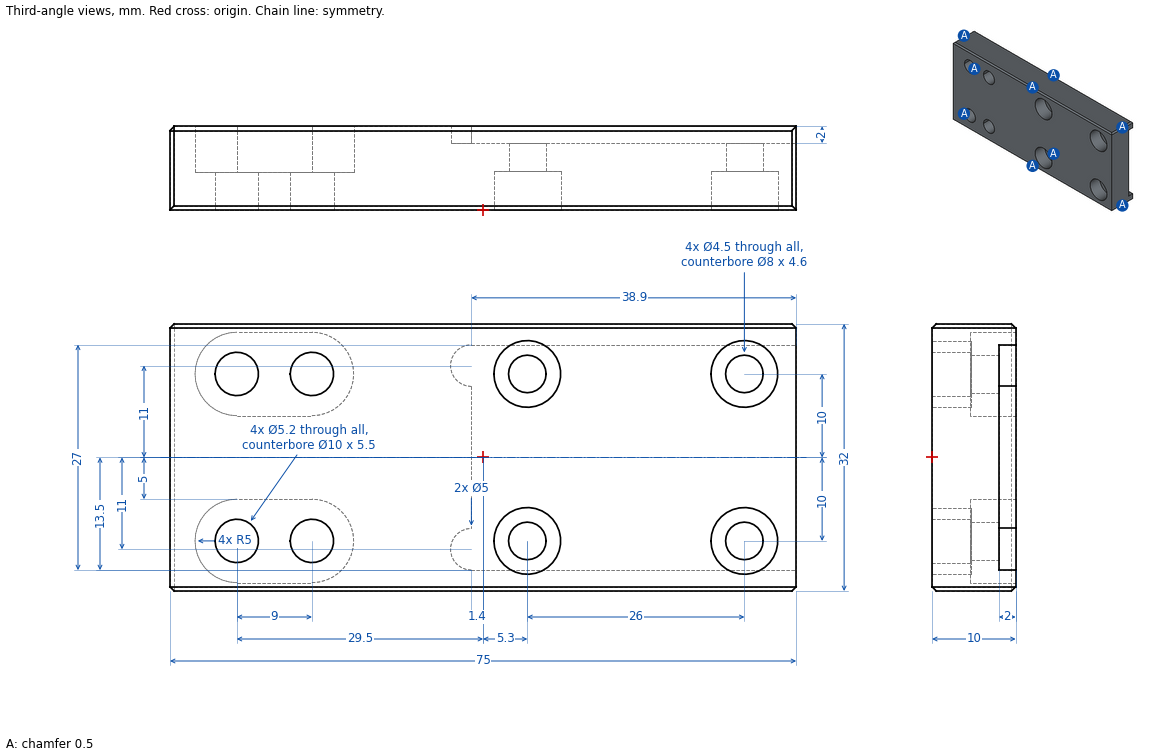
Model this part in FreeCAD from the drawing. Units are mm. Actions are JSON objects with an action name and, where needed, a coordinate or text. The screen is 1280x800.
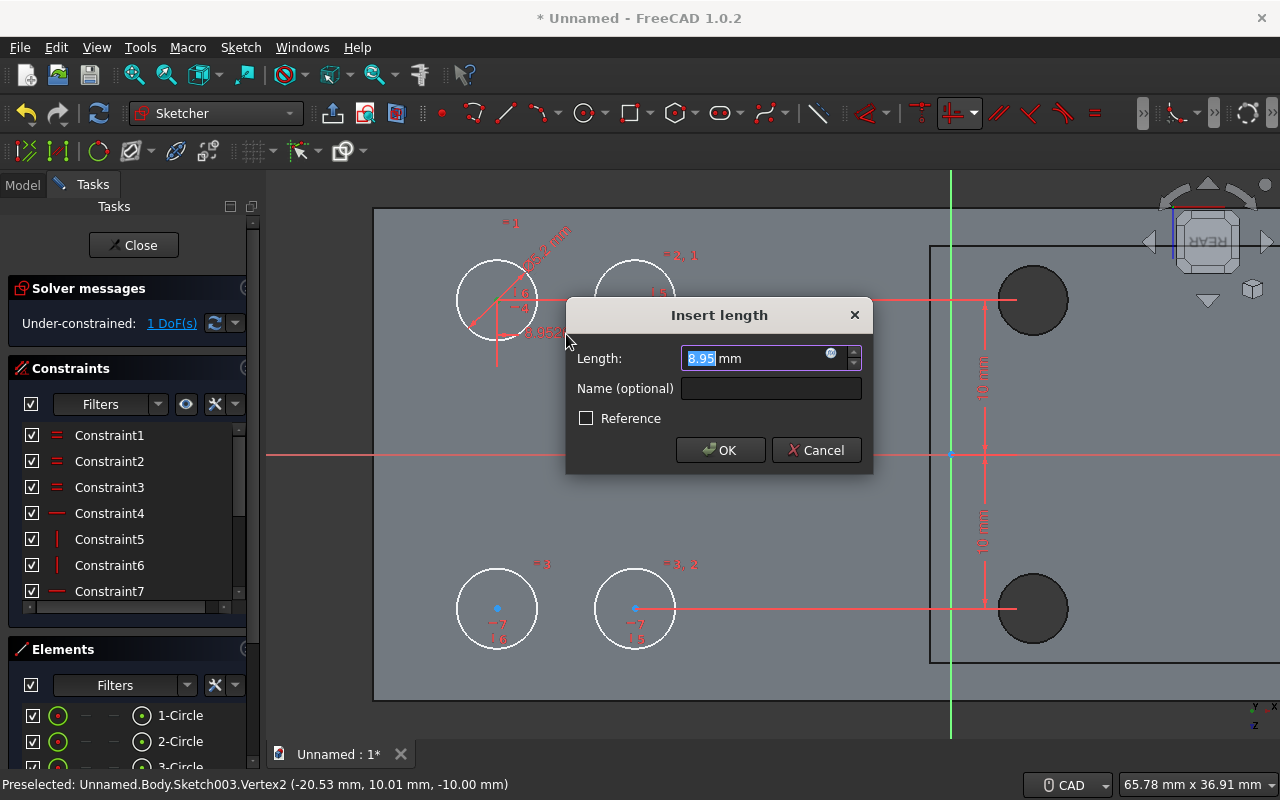
{"action": "type", "text": "9"}
{"action": "key", "text": "Return"}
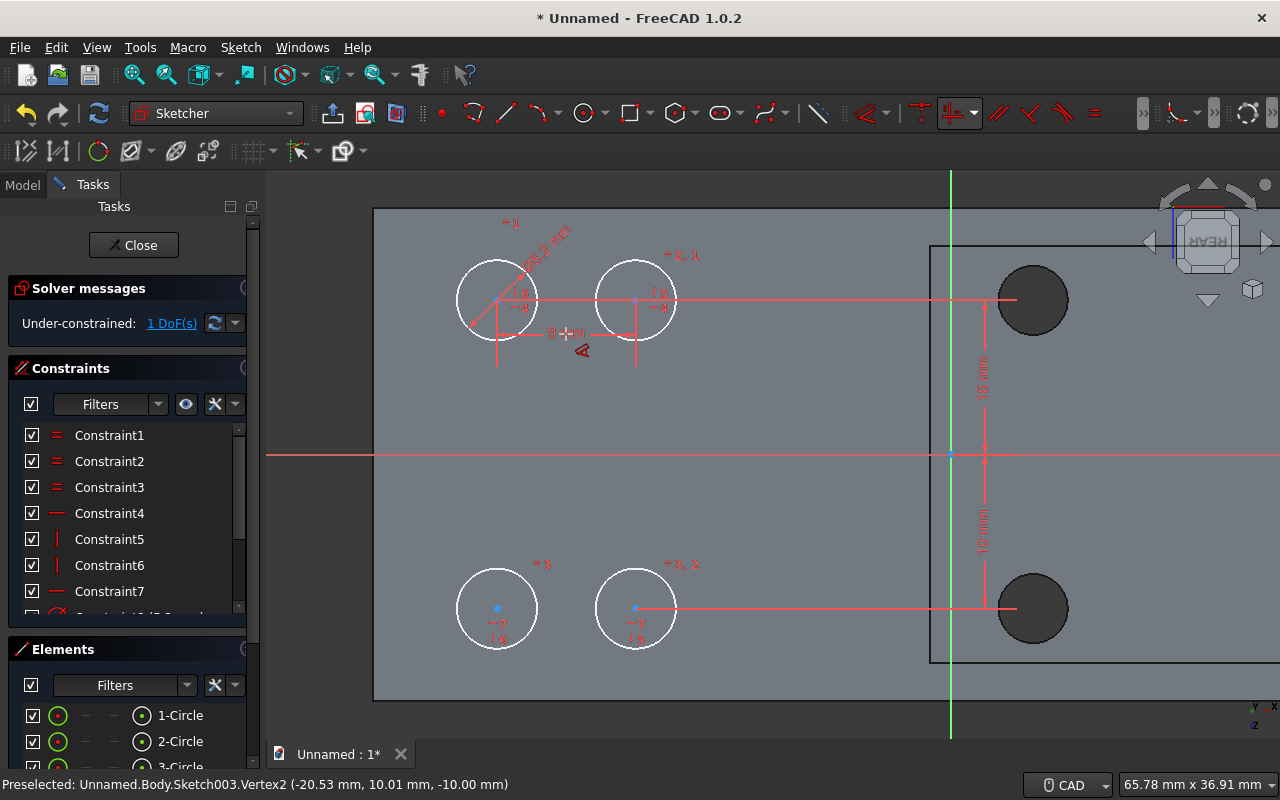
{"action": "left_click", "coordinate": [497, 300]}
{"action": "left_click", "coordinate": [724, 266]}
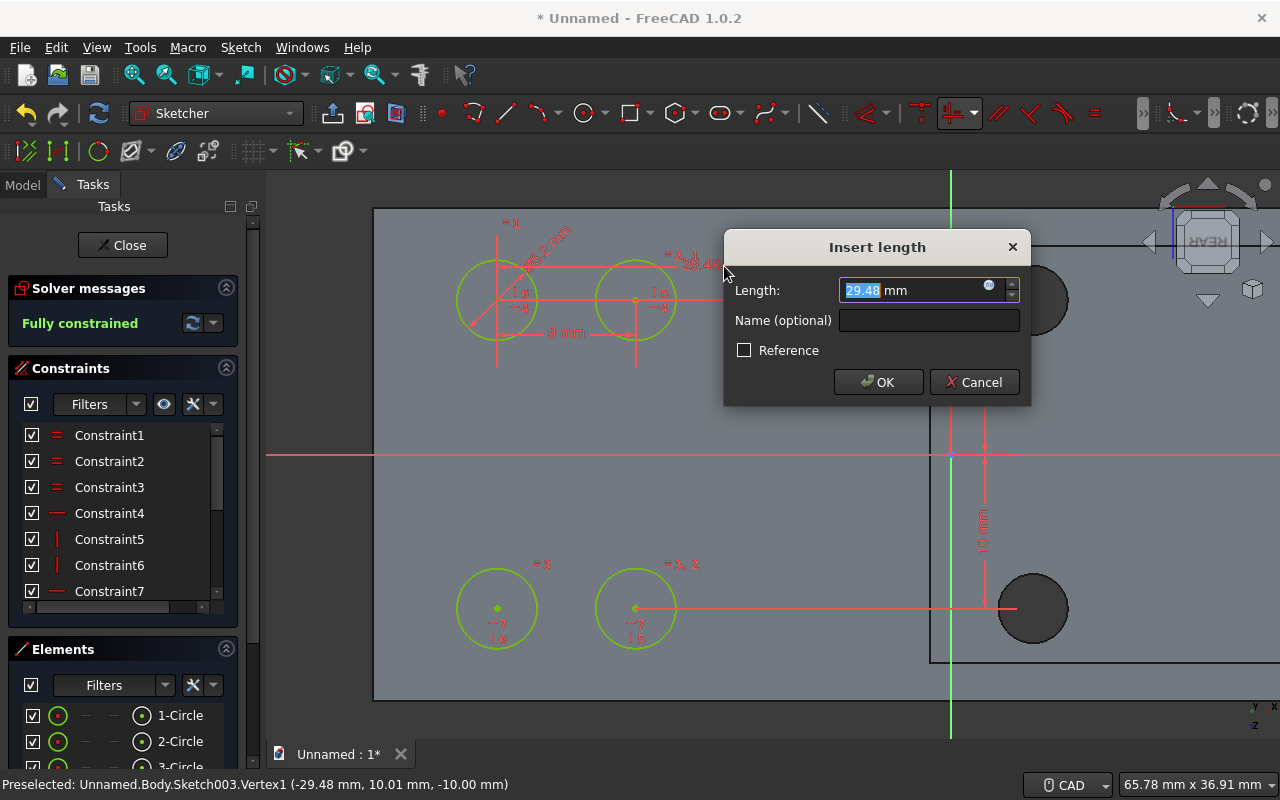
{"action": "type", "text": "29.5"}
{"action": "key", "text": "Return"}
{"action": "key", "text": "Escape"}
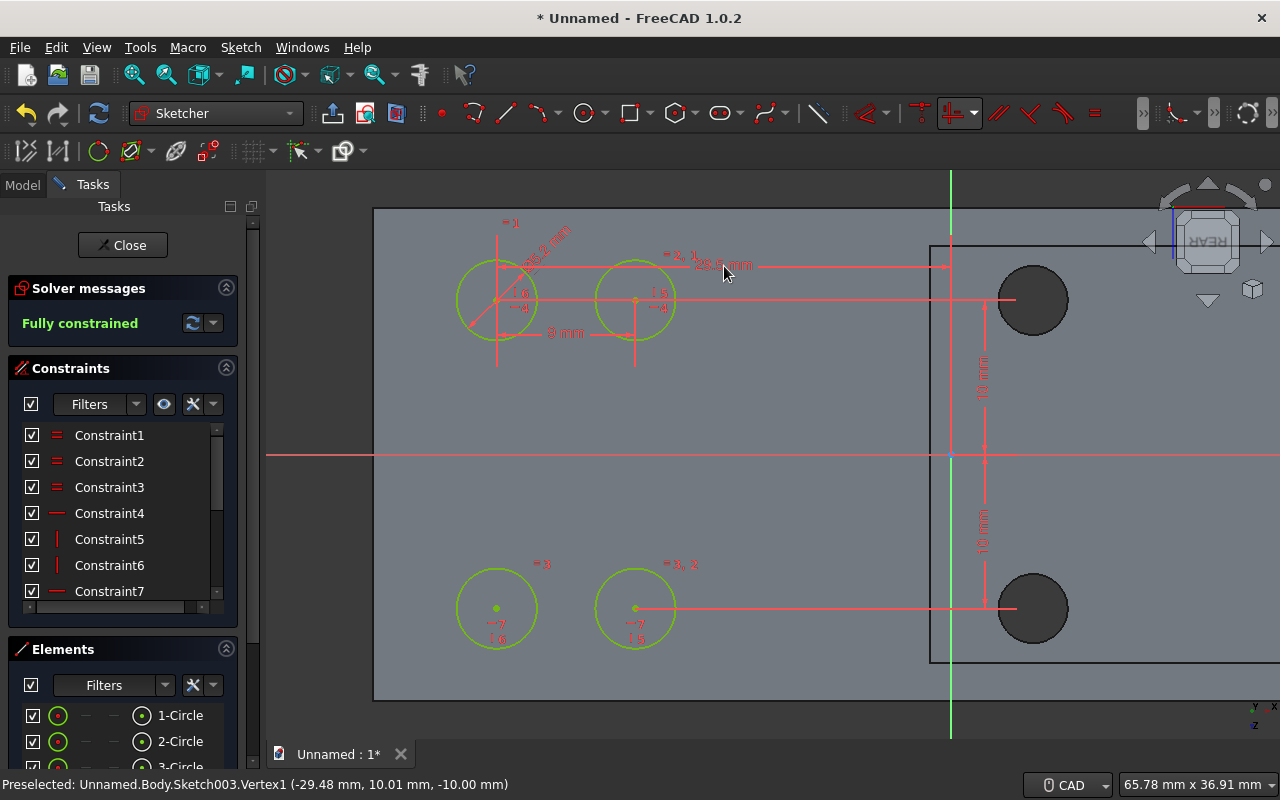
{"action": "left_click", "coordinate": [123, 245]}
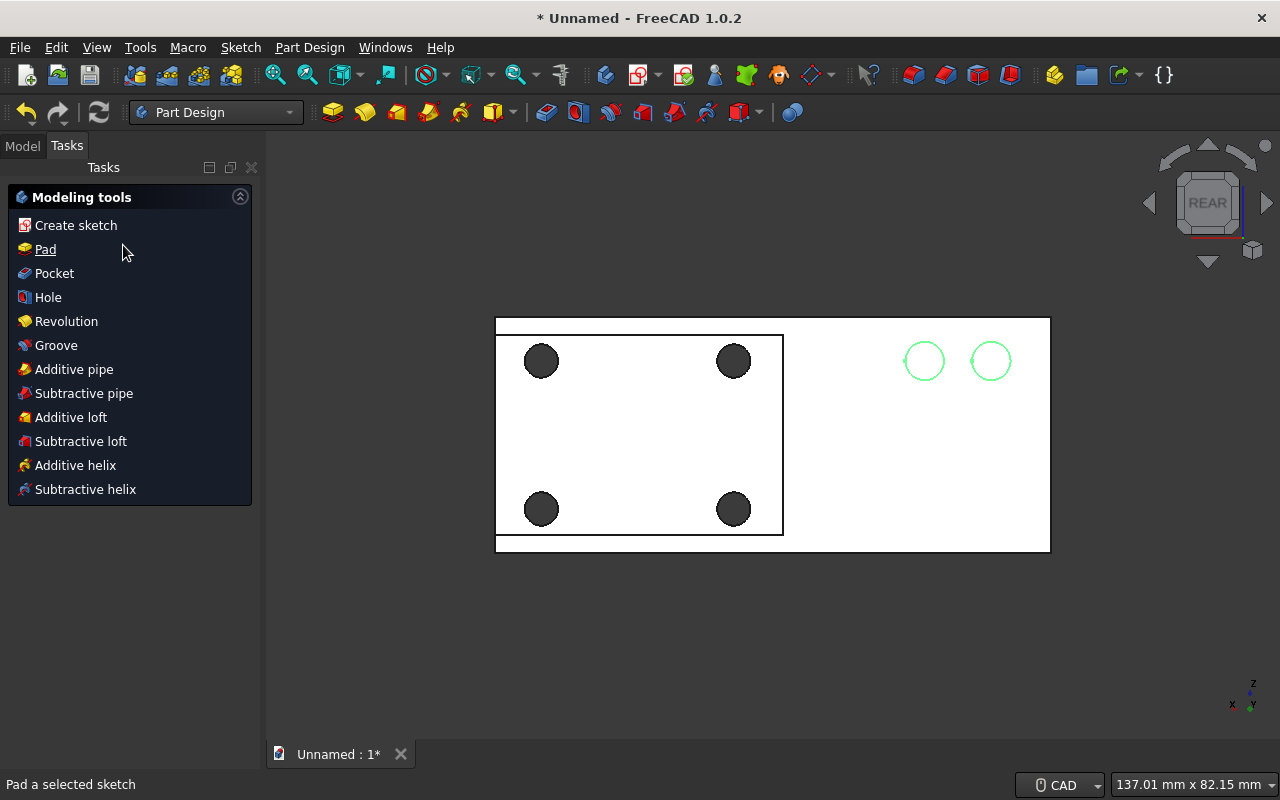
{"action": "left_click", "coordinate": [580, 112]}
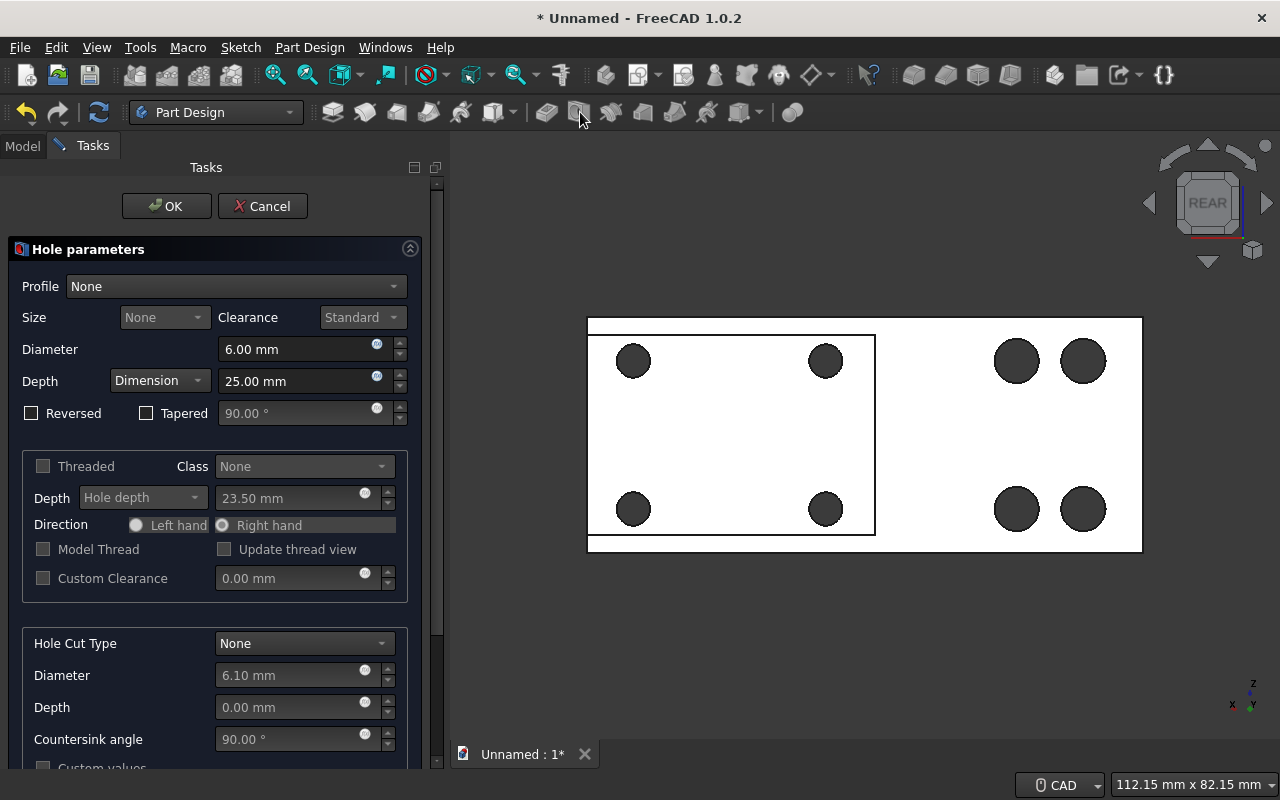
{"action": "triple_click", "coordinate": [305, 349]}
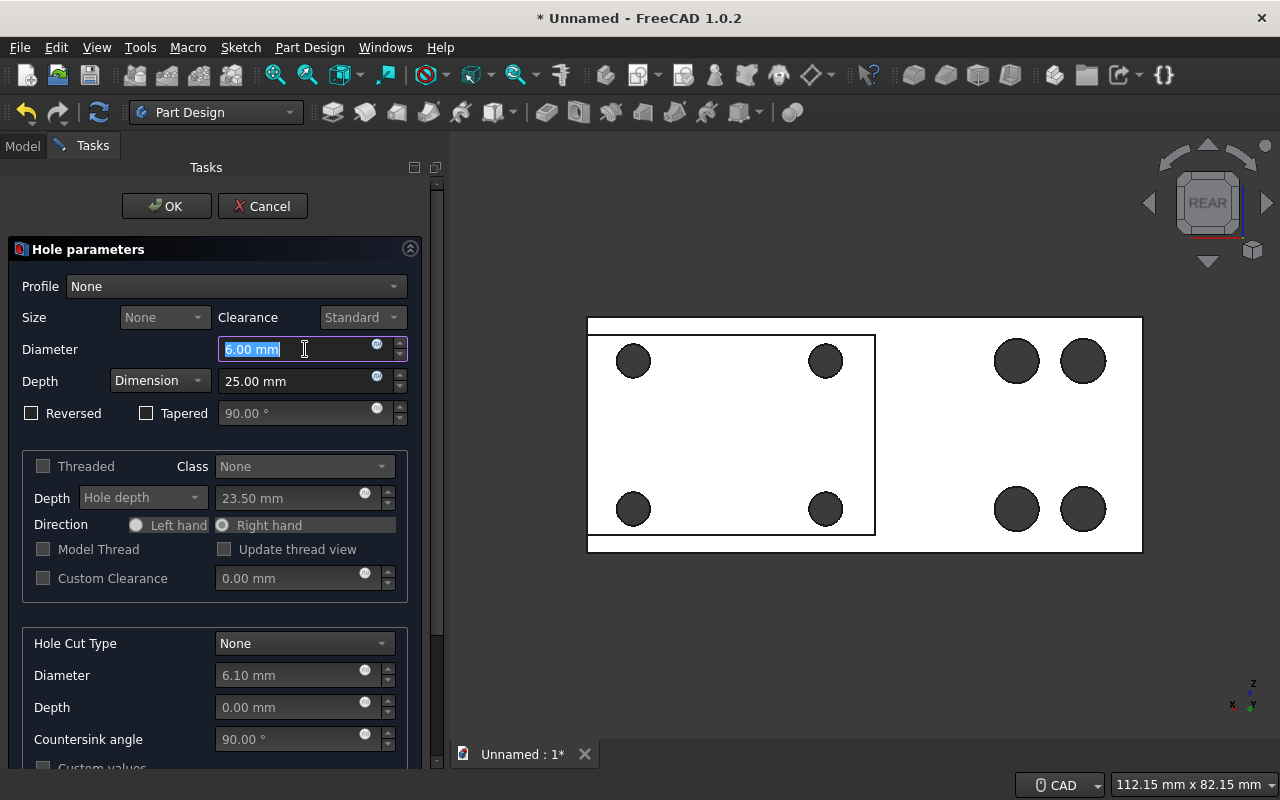
{"action": "type", "text": "5.2"}
{"action": "key", "text": "Tab"}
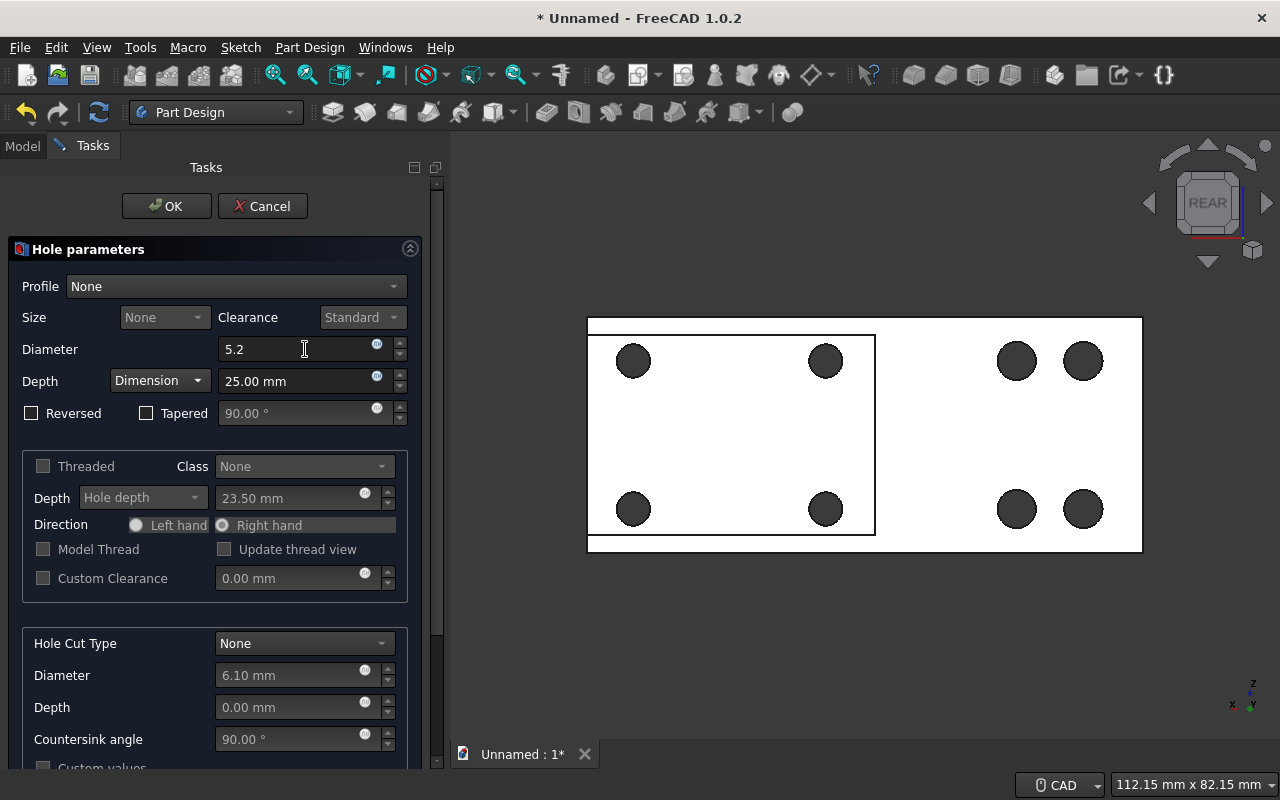
{"action": "left_click", "coordinate": [161, 380]}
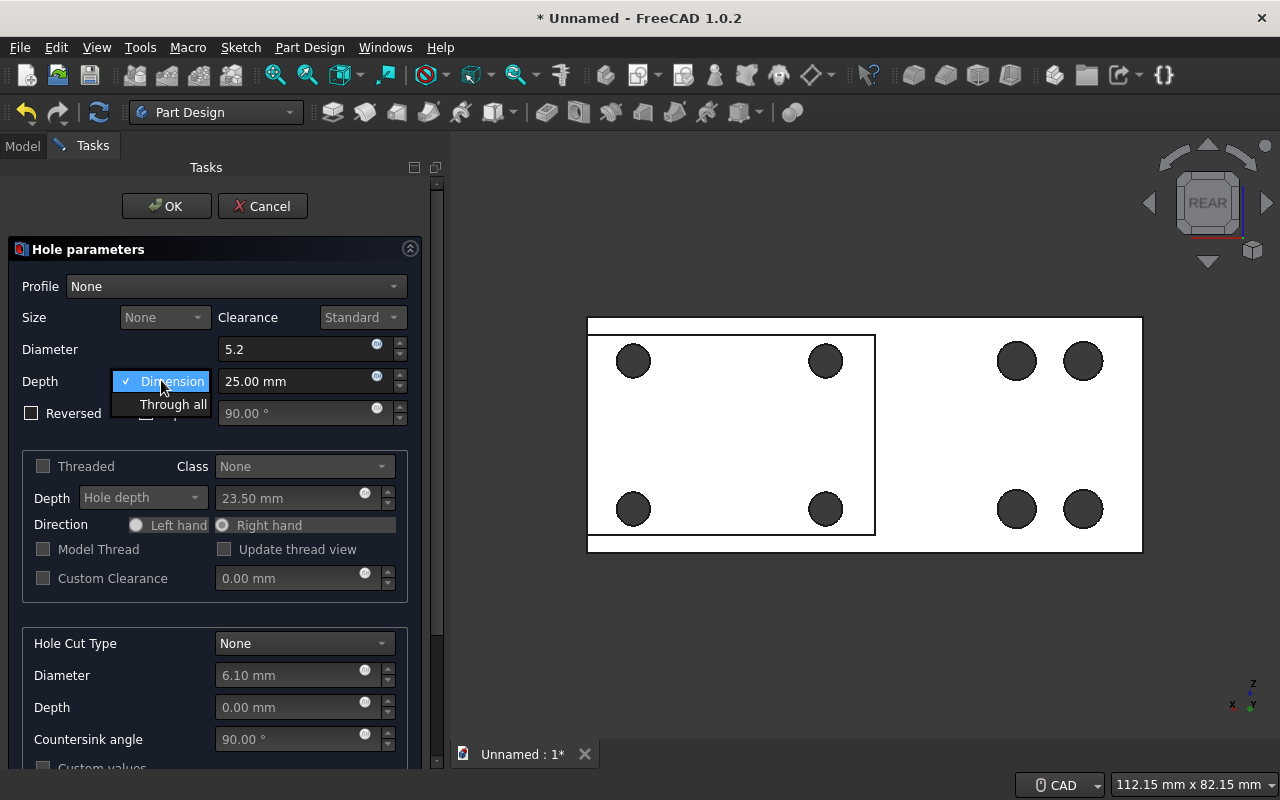
{"action": "left_click", "coordinate": [160, 404]}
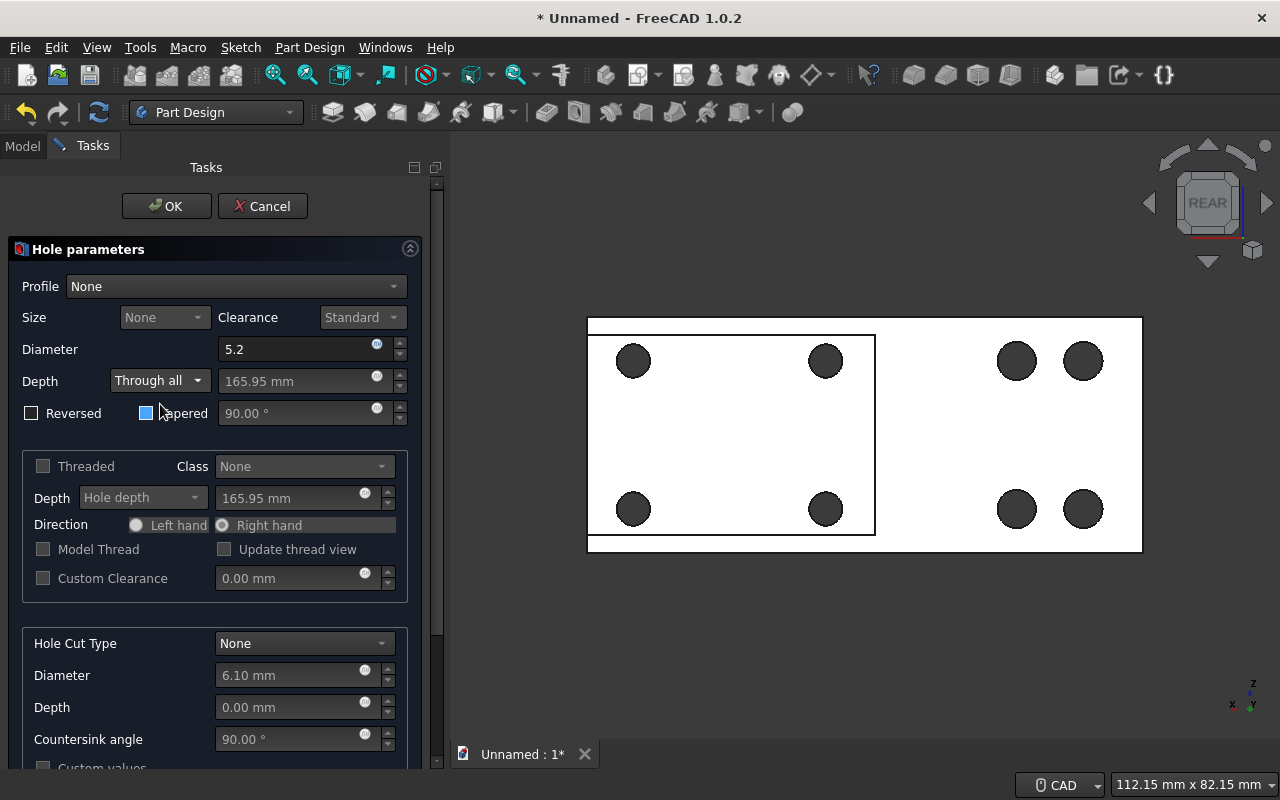
{"action": "left_click", "coordinate": [306, 644]}